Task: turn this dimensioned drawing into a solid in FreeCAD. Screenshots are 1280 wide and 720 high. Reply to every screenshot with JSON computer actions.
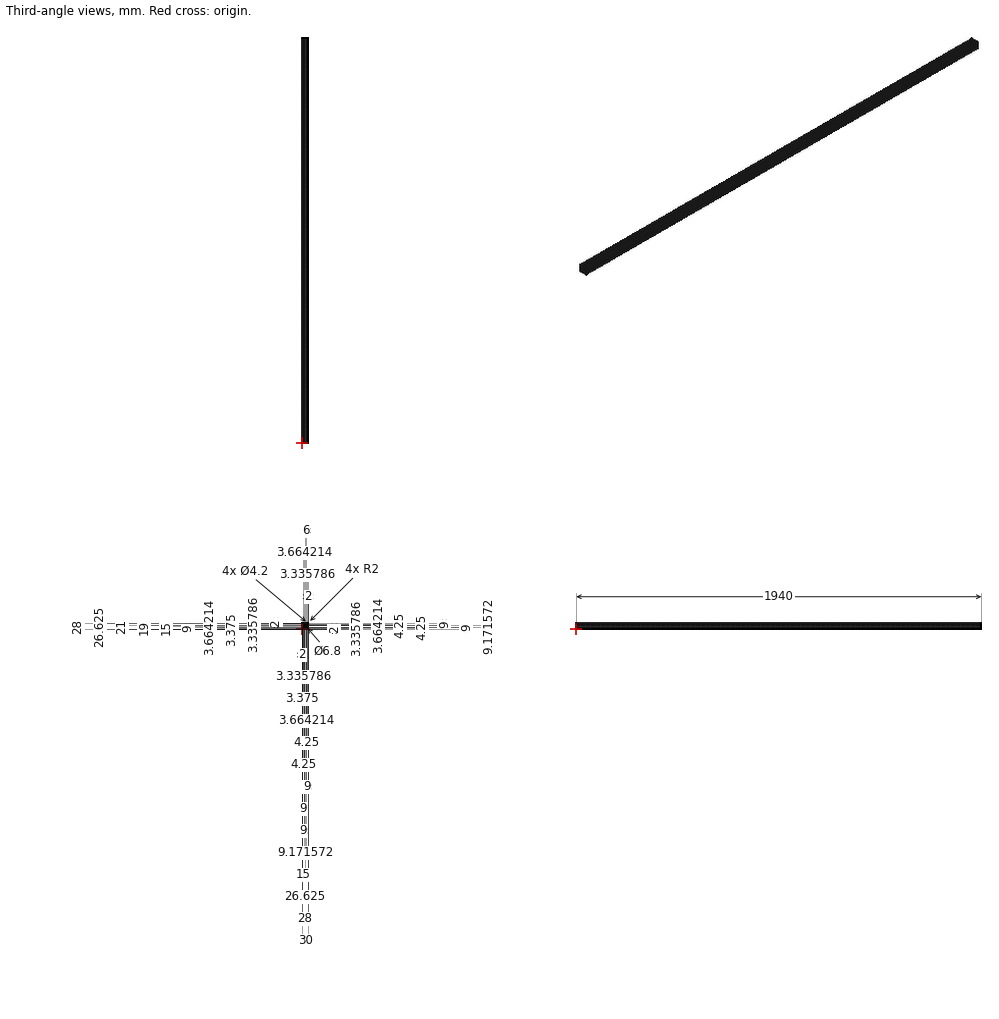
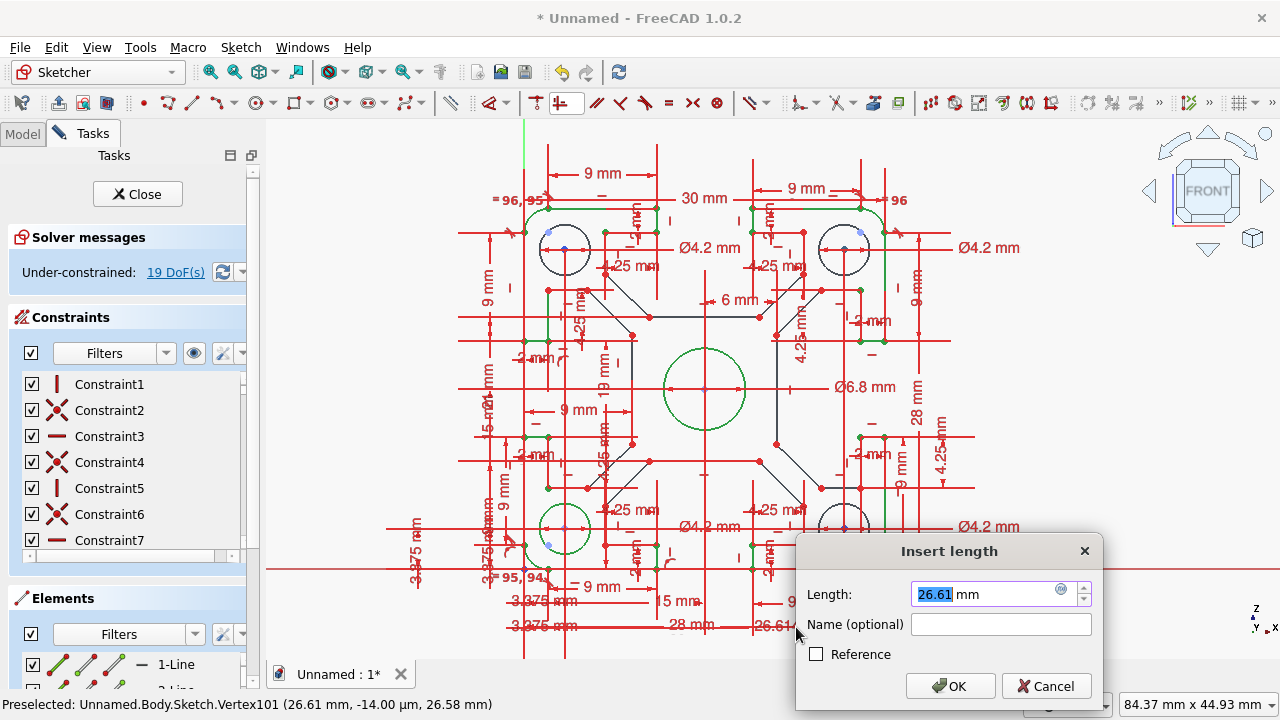
{"action": "type", "text": "26.625"}
{"action": "key", "text": "Return"}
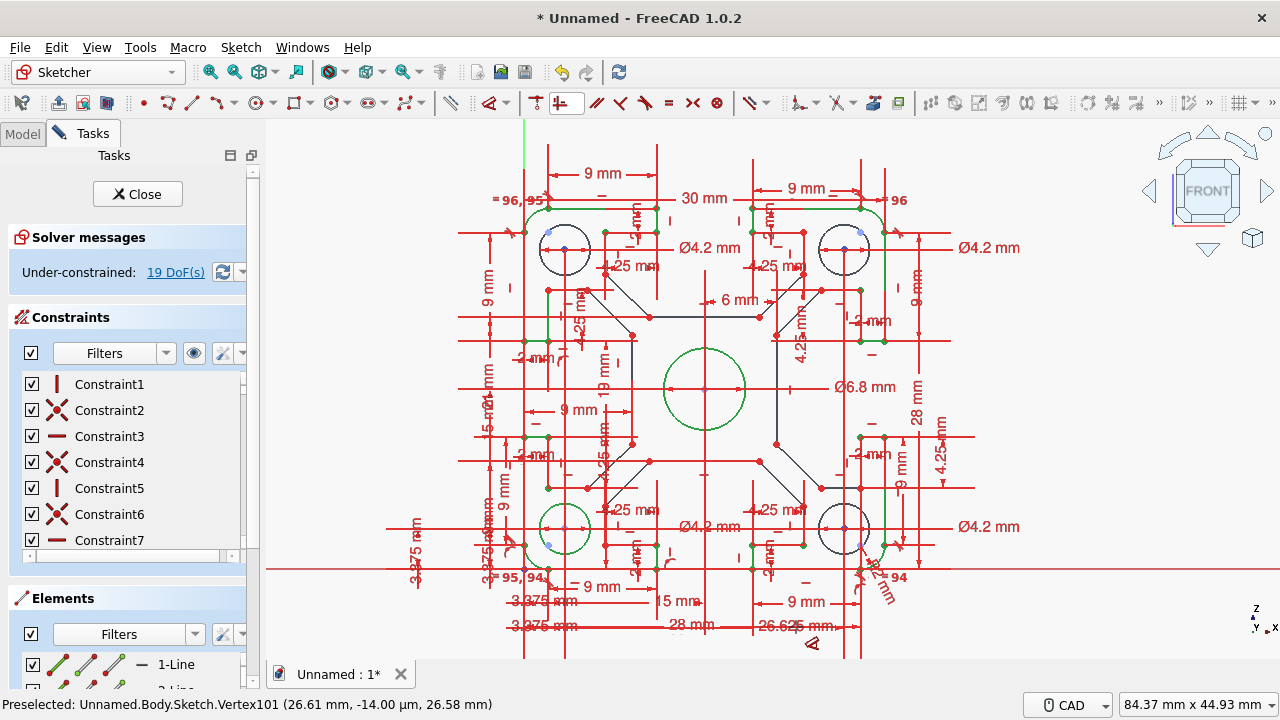
{"action": "left_click", "coordinate": [844, 250]}
{"action": "left_click", "coordinate": [490, 336]}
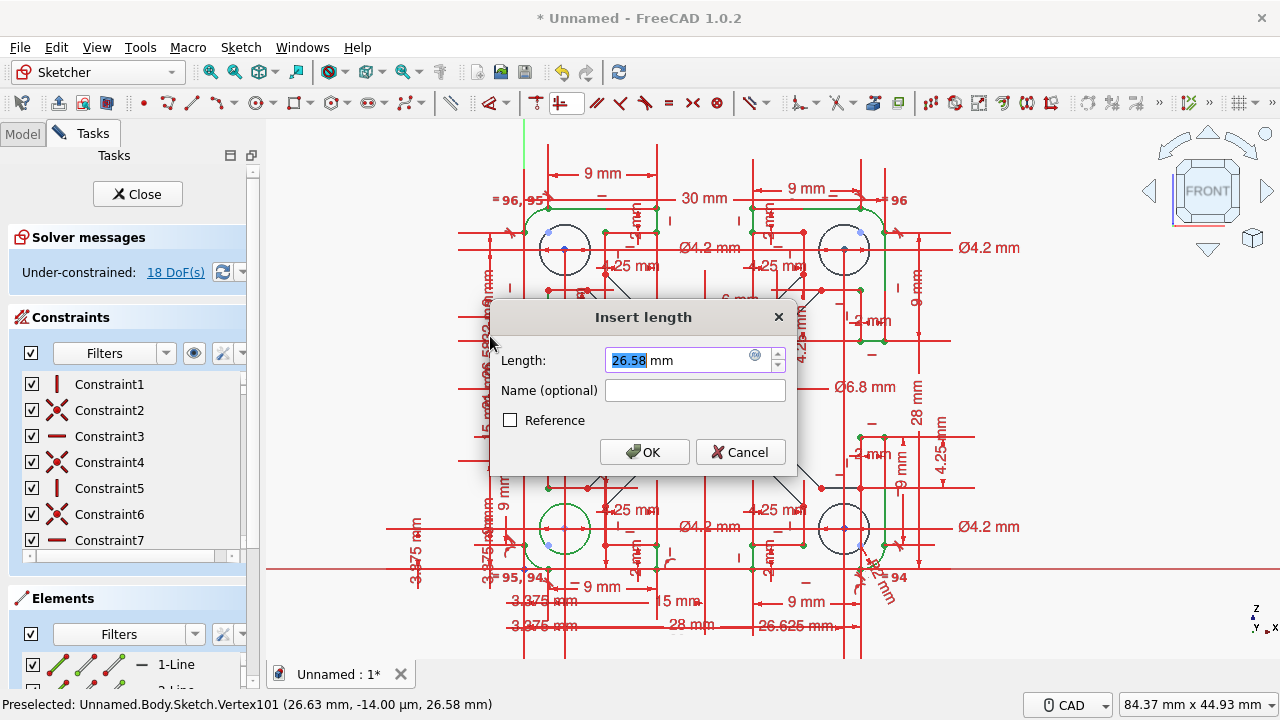
{"action": "type", "text": "26.625"}
{"action": "key", "text": "Return"}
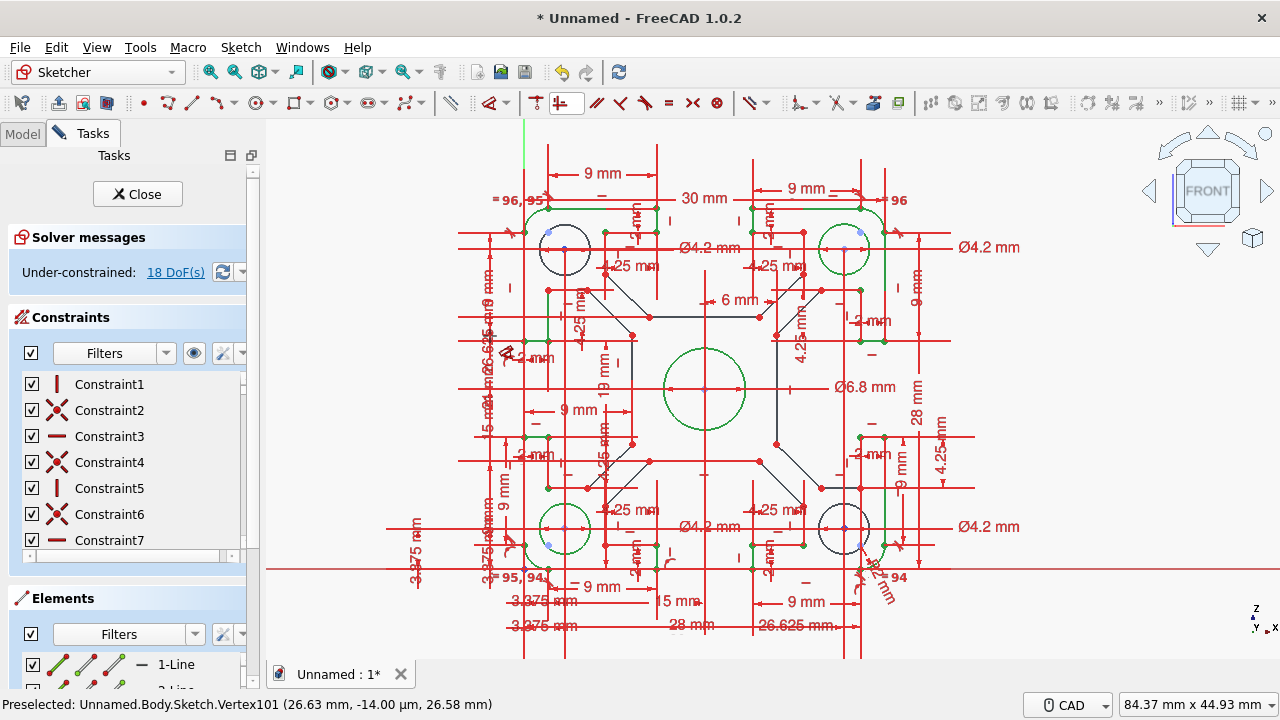
{"action": "left_click", "coordinate": [565, 250]}
{"action": "left_click", "coordinate": [599, 336]}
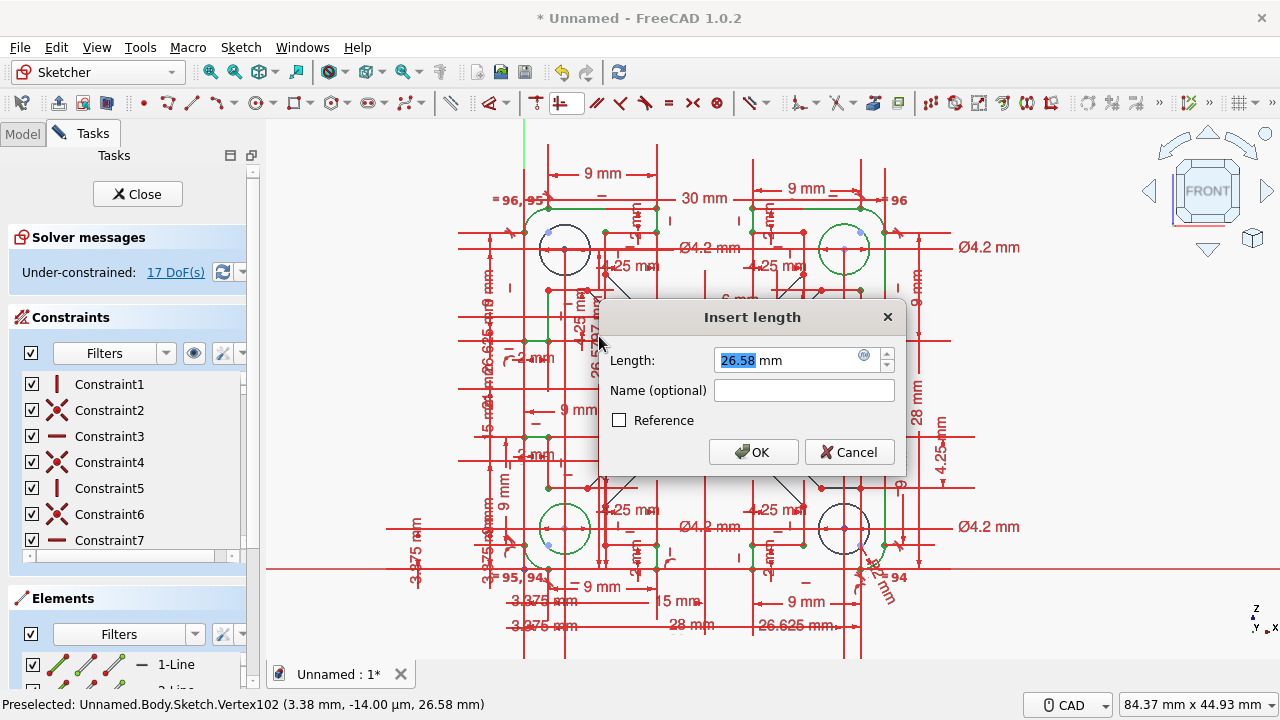
{"action": "type", "text": "26.625"}
{"action": "key", "text": "Return"}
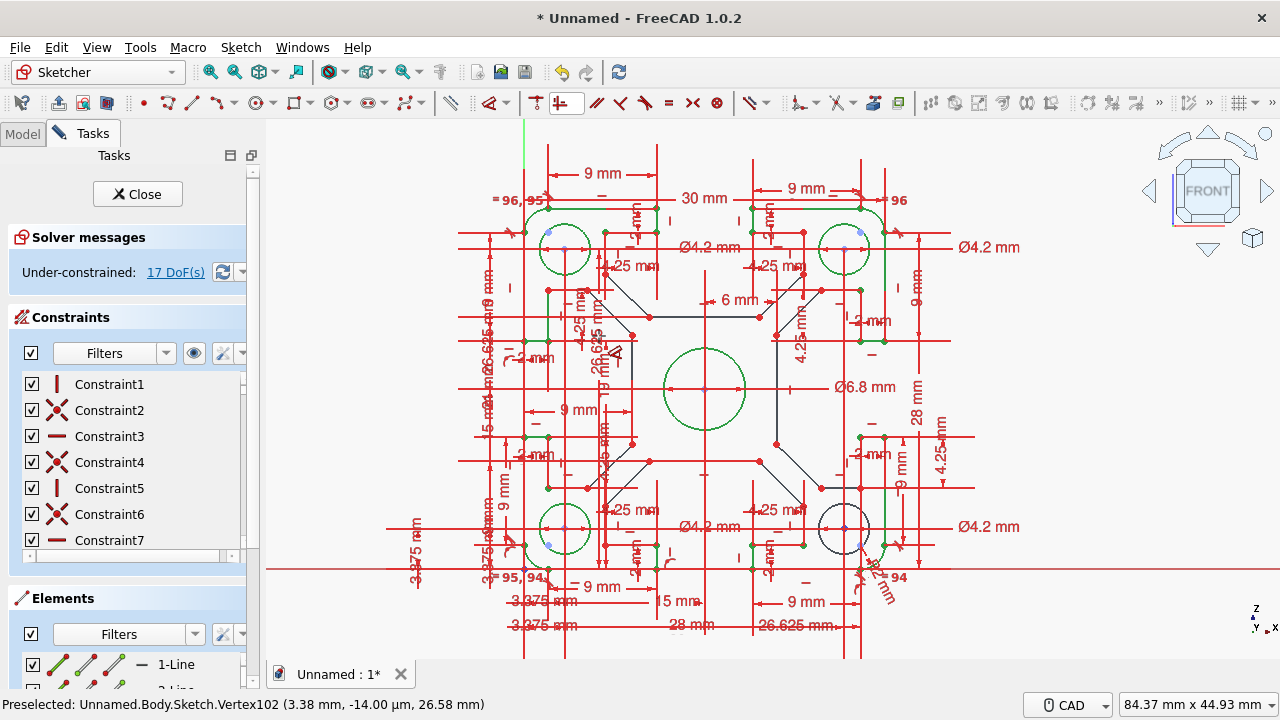
{"action": "left_click", "coordinate": [844, 529]}
{"action": "left_click", "coordinate": [684, 447]}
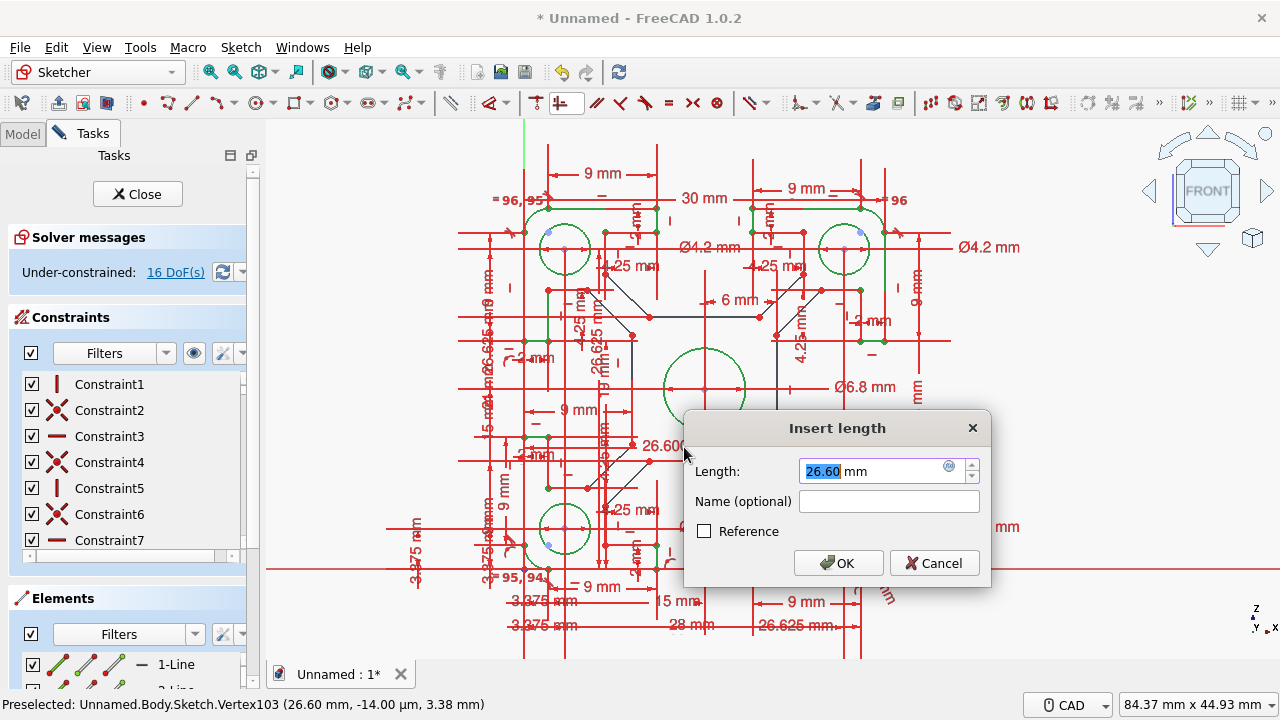
{"action": "type", "text": "26.625"}
{"action": "key", "text": "Return"}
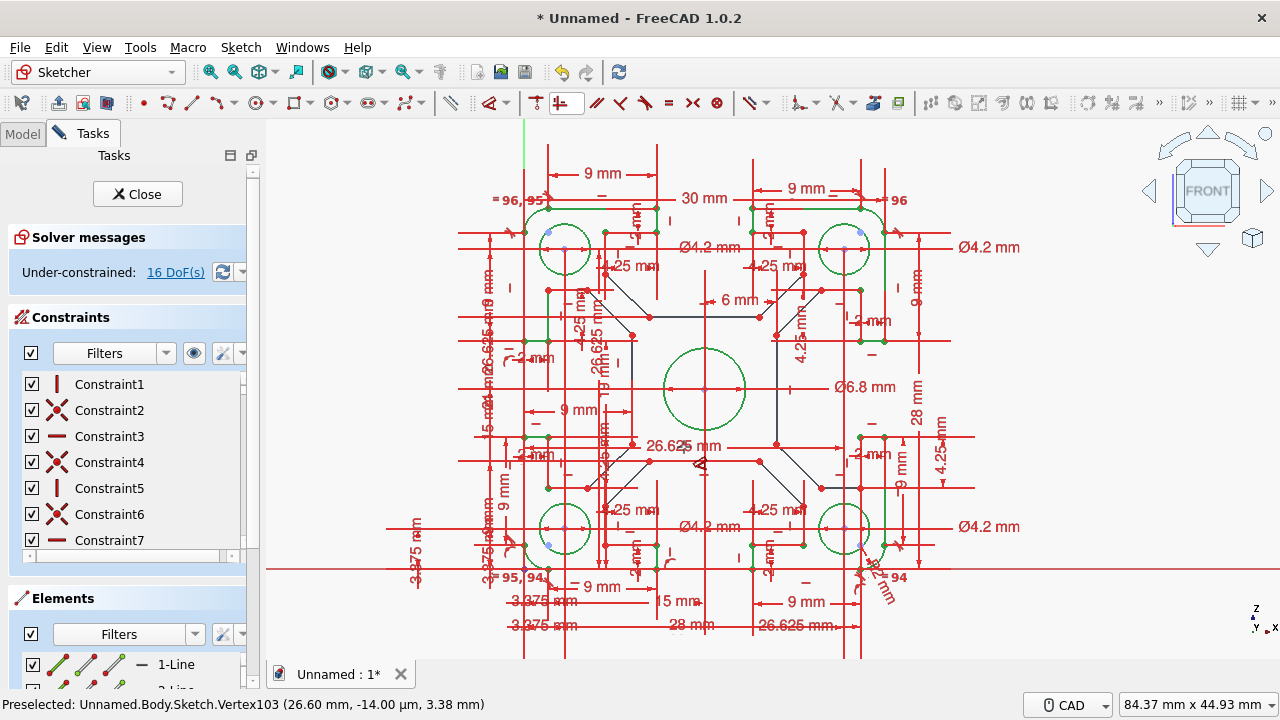
{"action": "left_click", "coordinate": [849, 290]}
{"action": "left_click", "coordinate": [850, 256]}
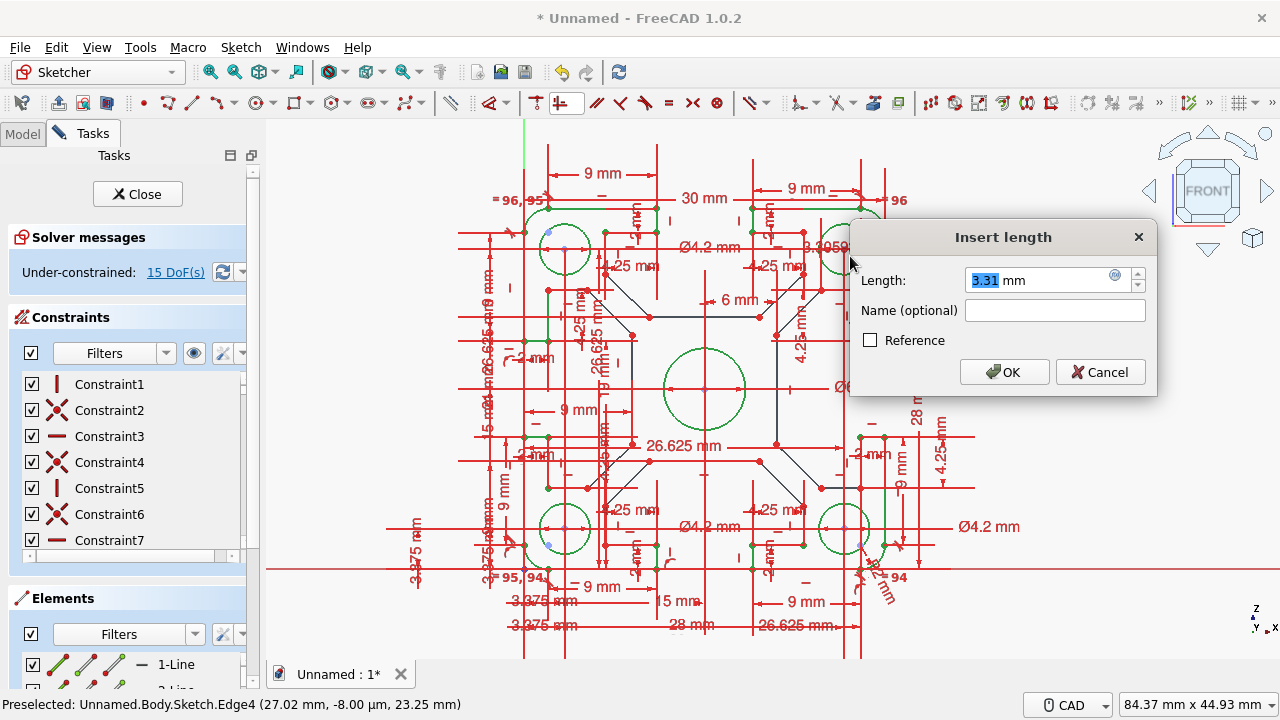
{"action": "type", "text": "3.335786"}
{"action": "key", "text": "Return"}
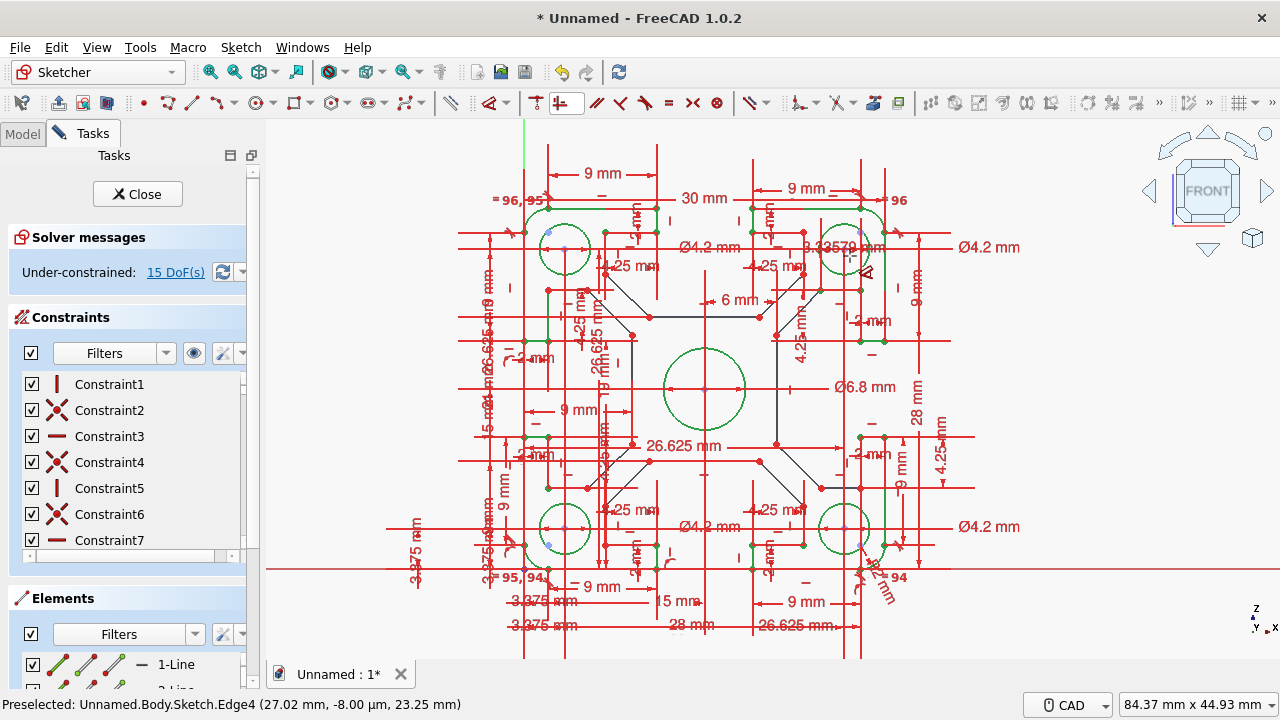
{"action": "left_click", "coordinate": [777, 368]}
{"action": "left_click", "coordinate": [811, 390]}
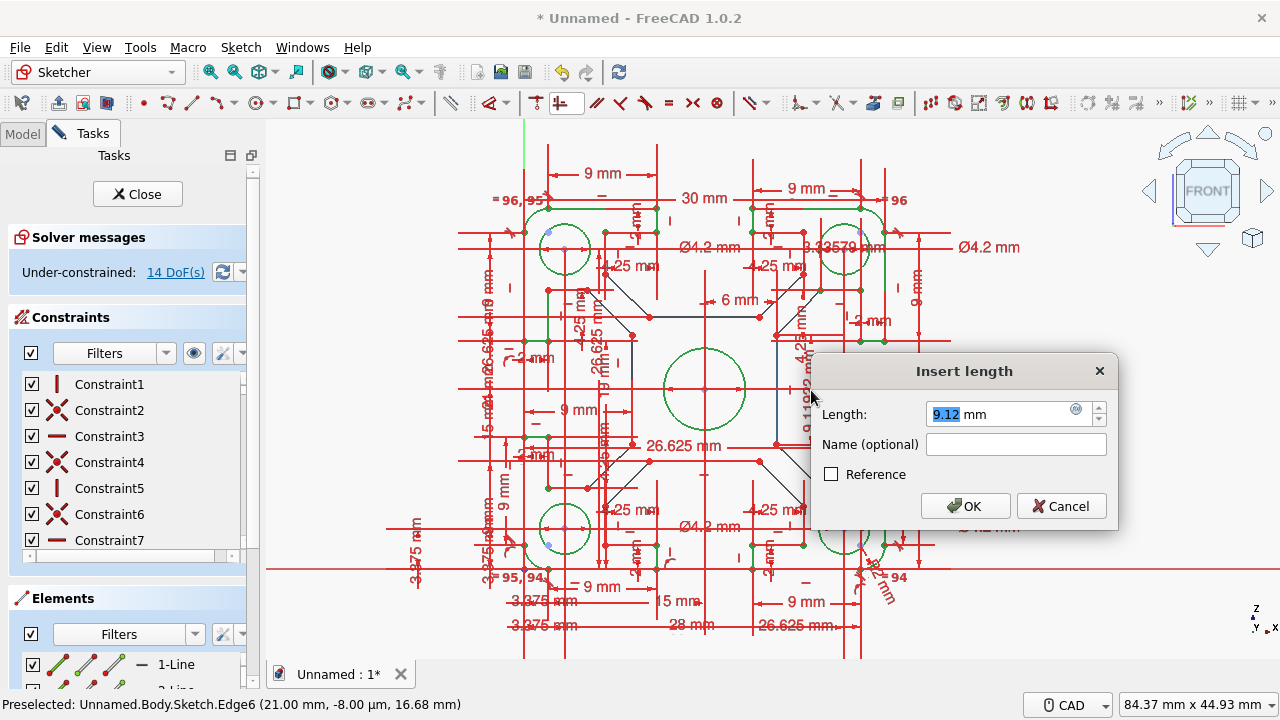
{"action": "type", "text": "9.171572"}
{"action": "key", "text": "Return"}